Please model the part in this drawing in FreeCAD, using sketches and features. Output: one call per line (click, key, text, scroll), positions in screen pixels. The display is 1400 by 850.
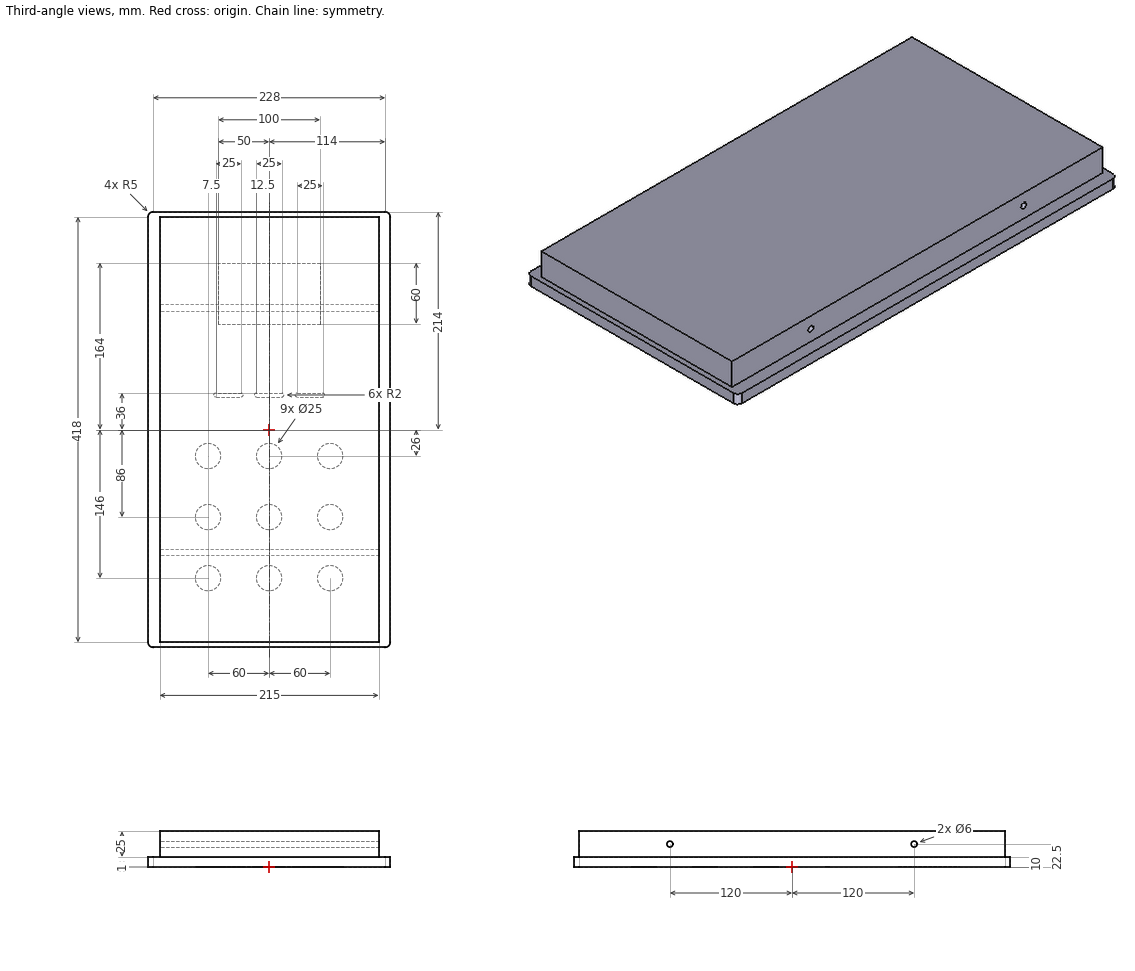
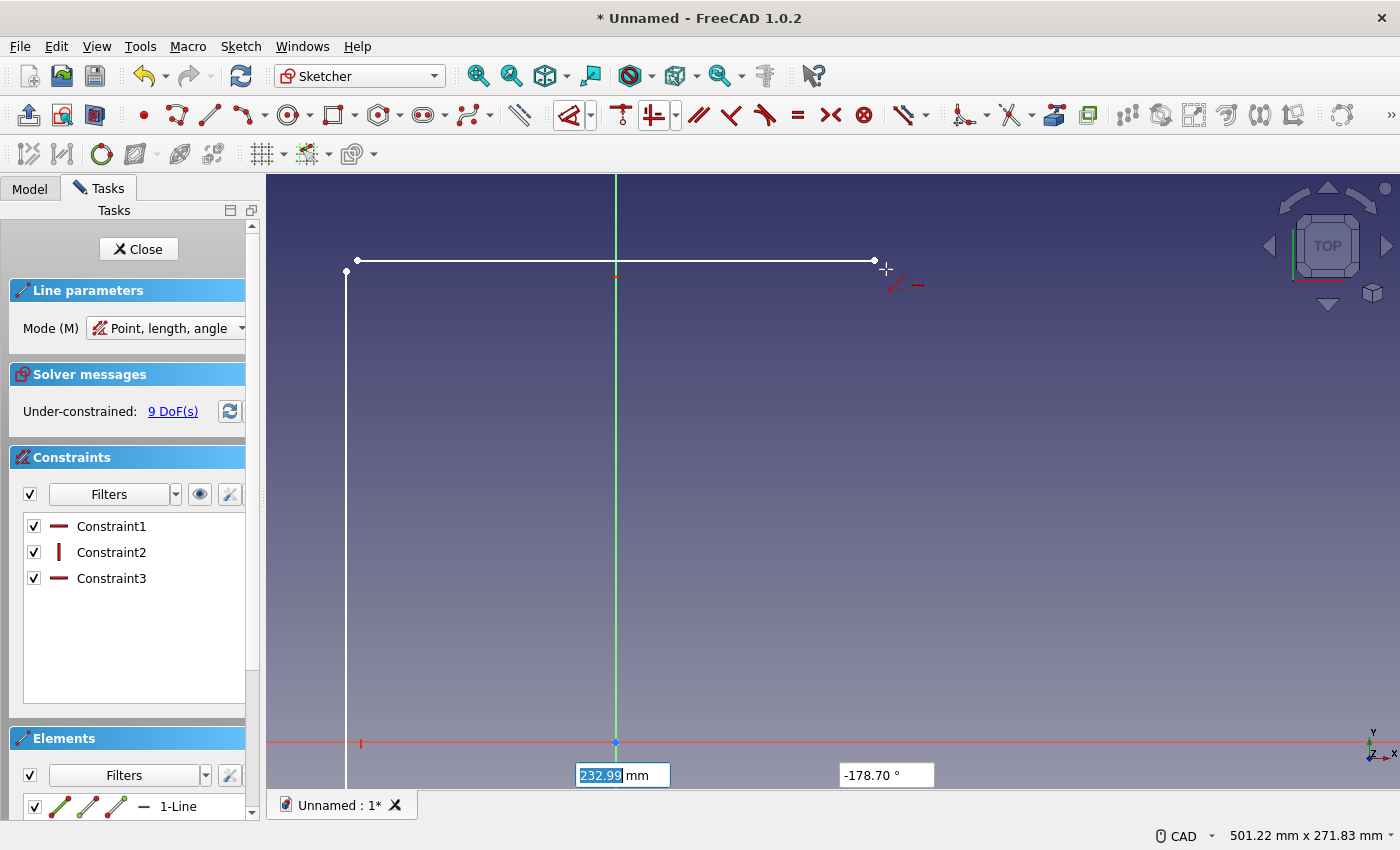
click(885, 270)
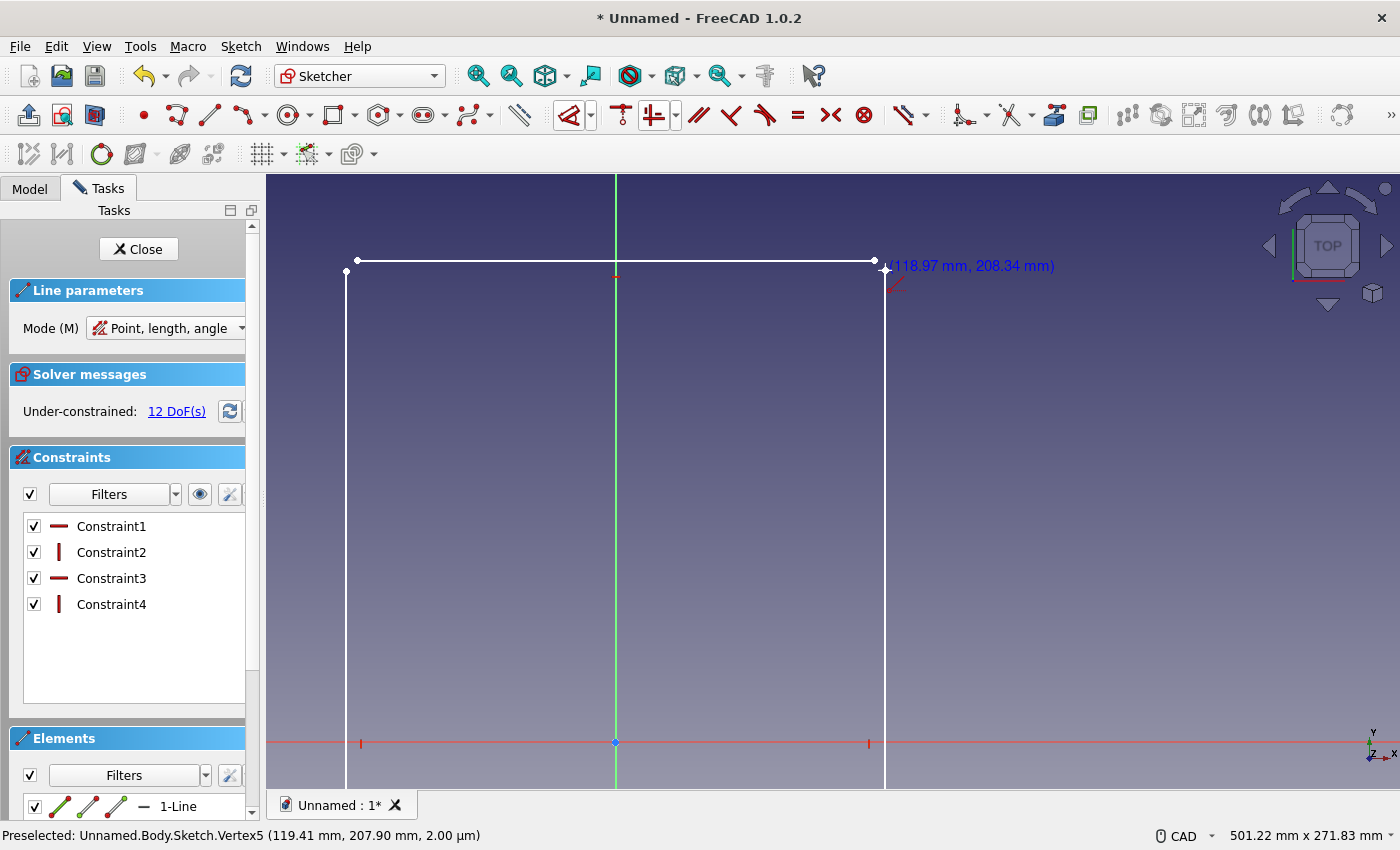
key(g)
key(3)
key(a)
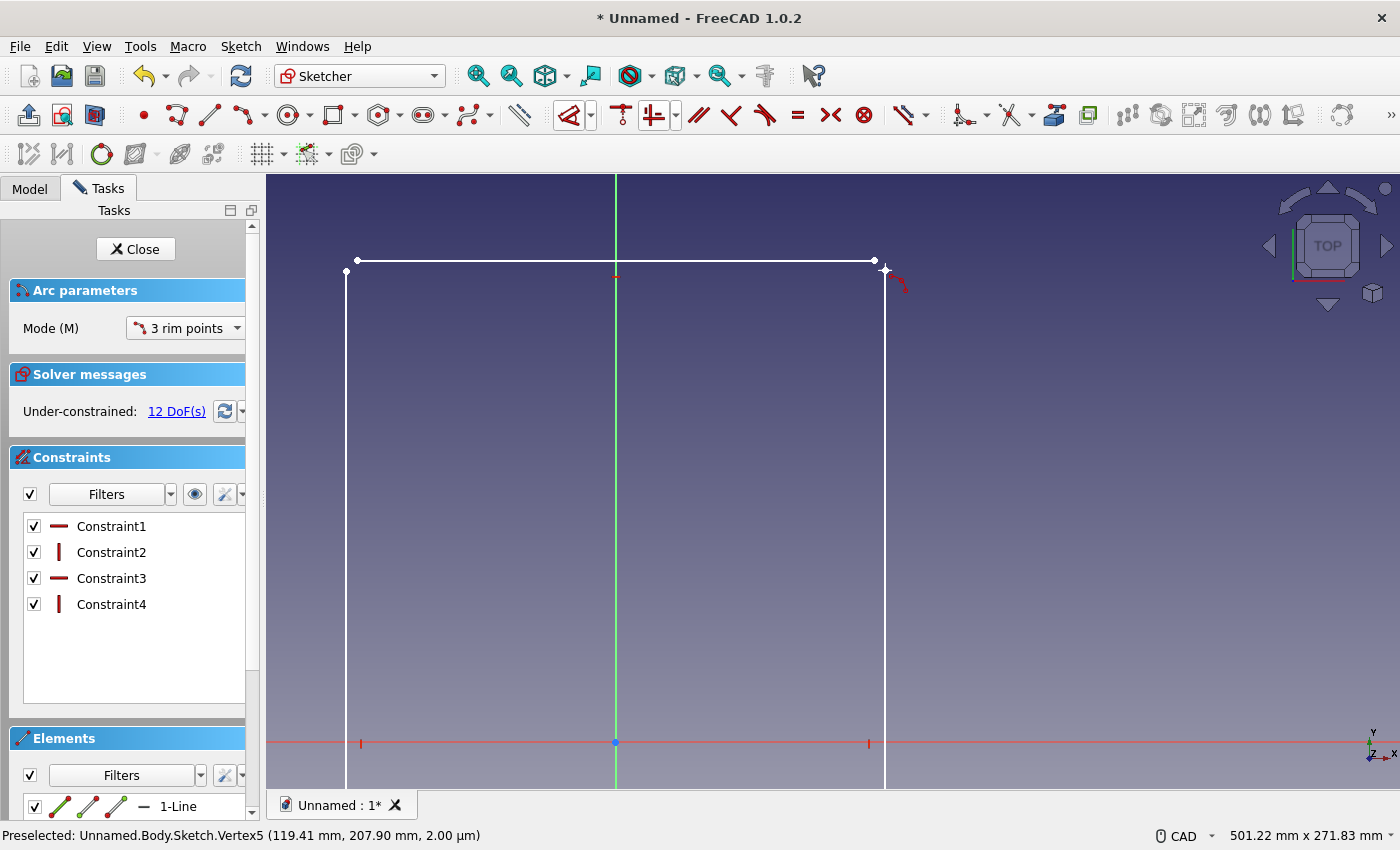
click(358, 261)
click(346, 271)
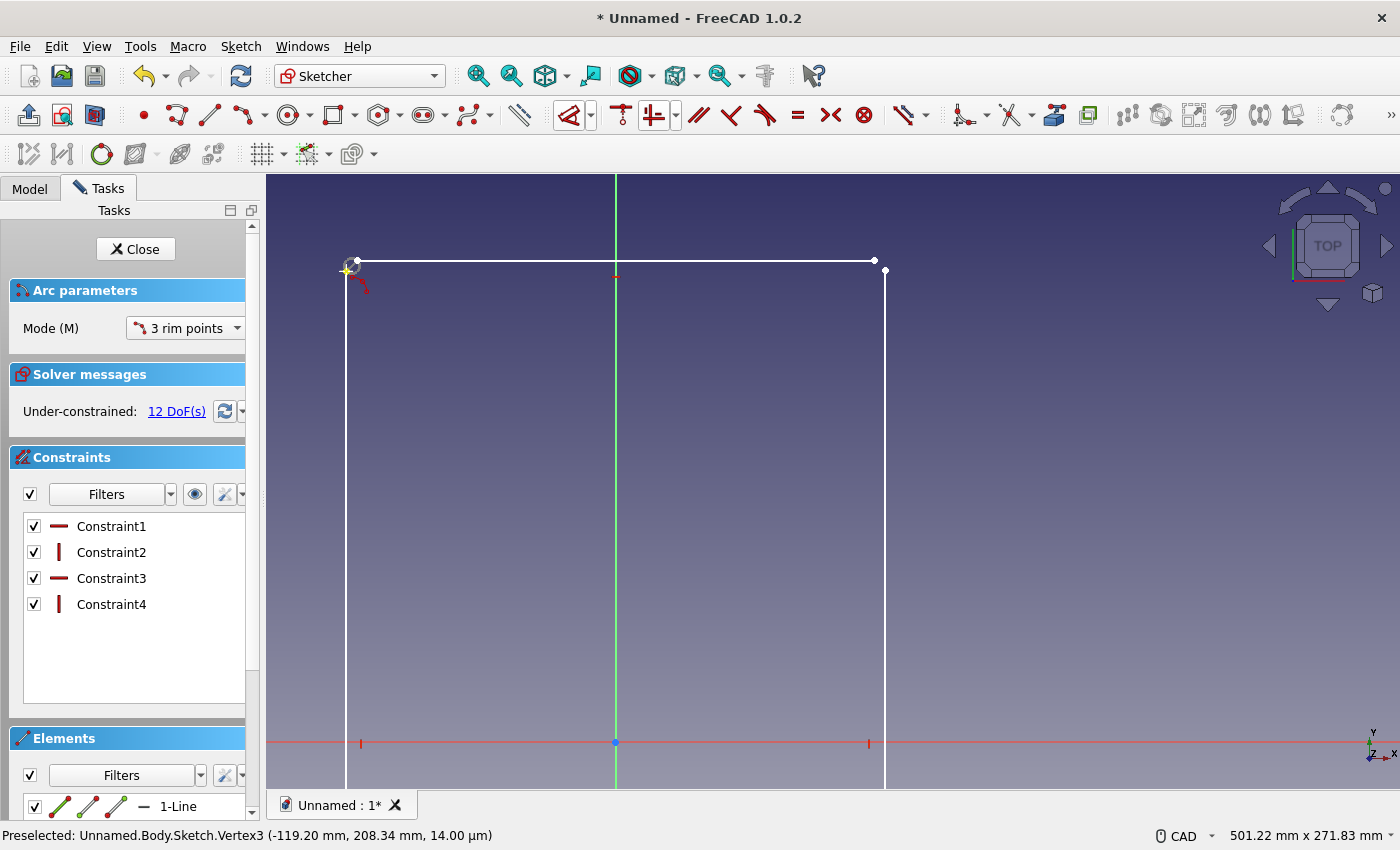
scroll(350, 262, up, 8)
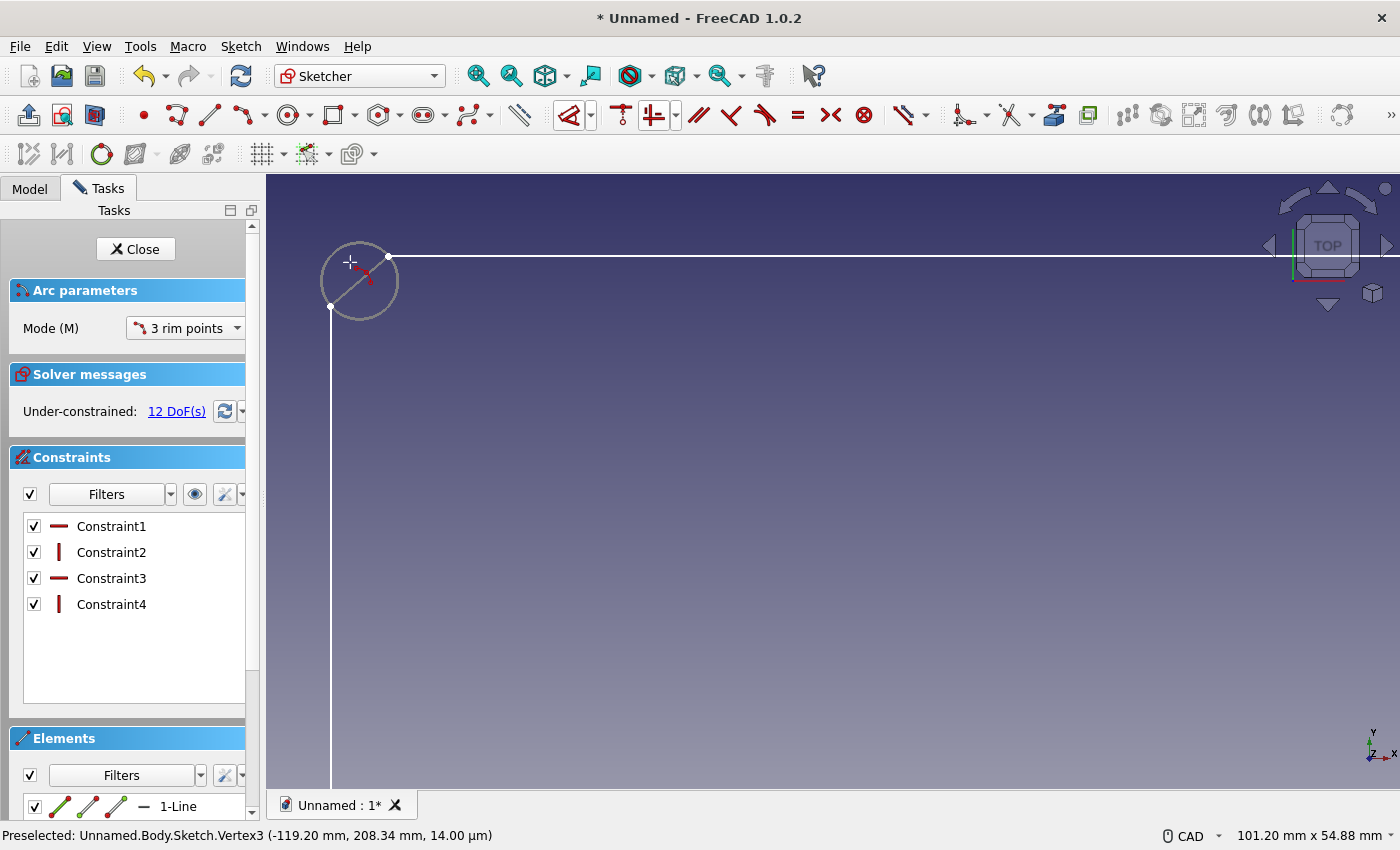
click(349, 259)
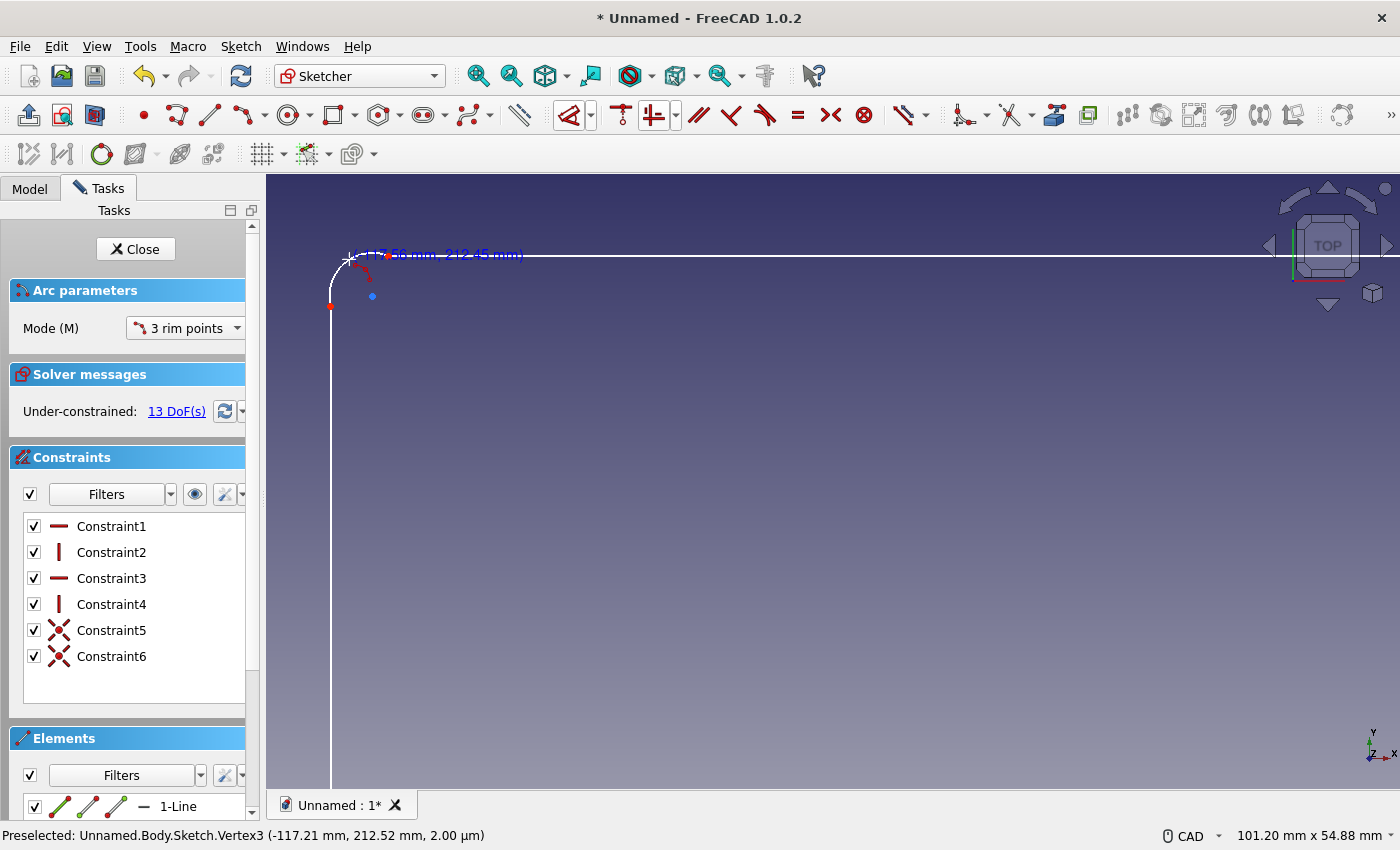
scroll(675, 266, down, 12)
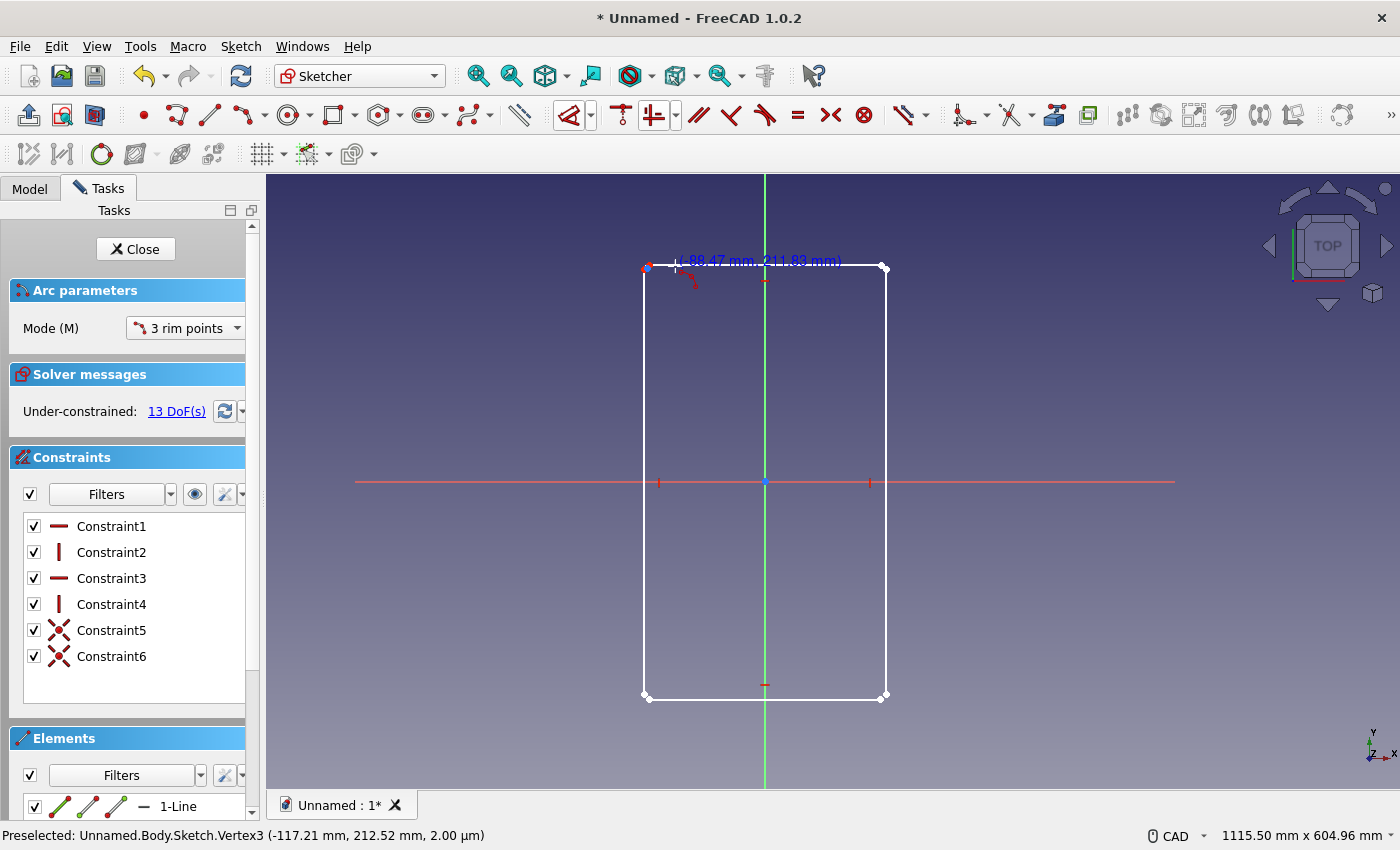
scroll(644, 694, up, 4)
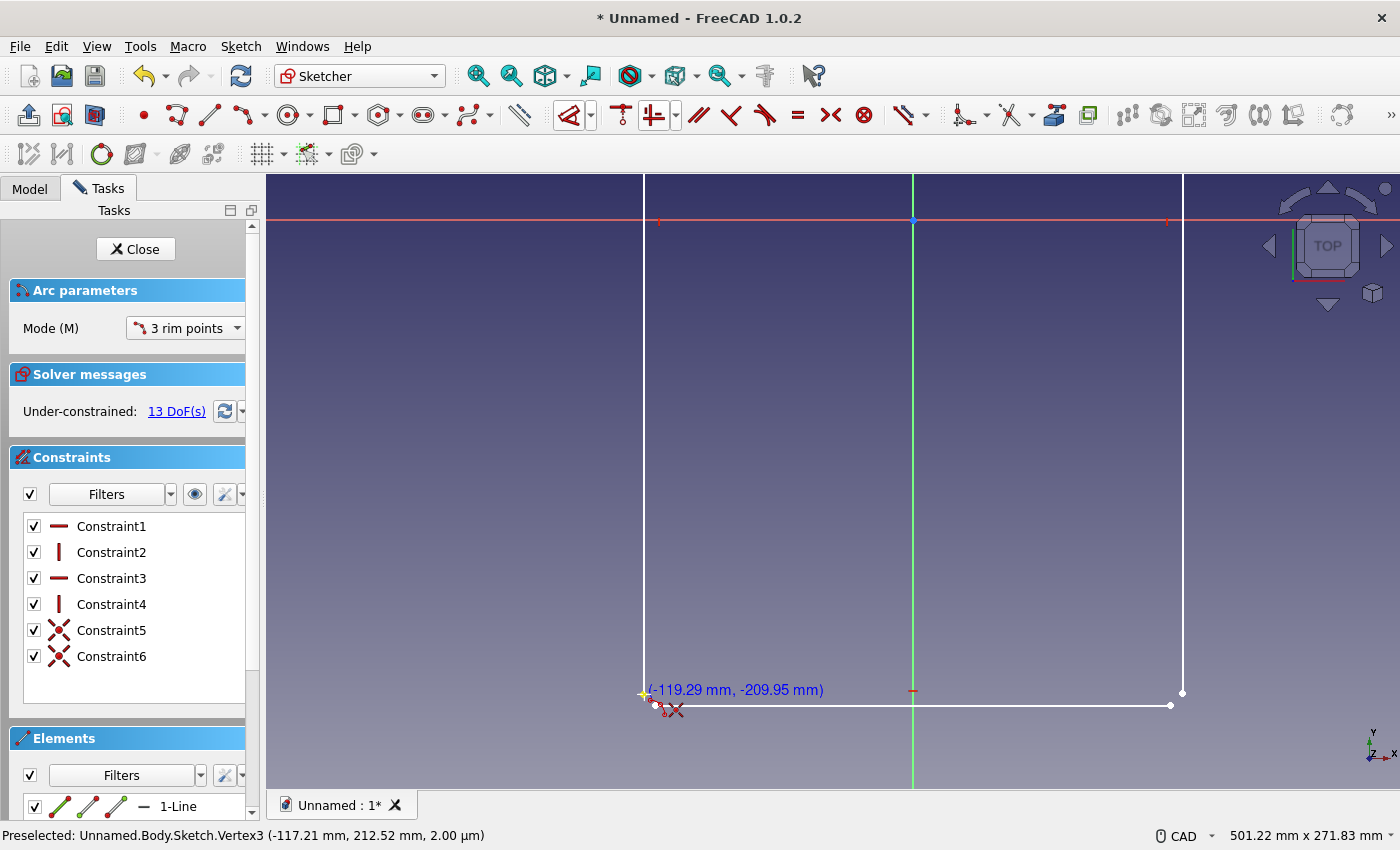
click(644, 695)
click(656, 706)